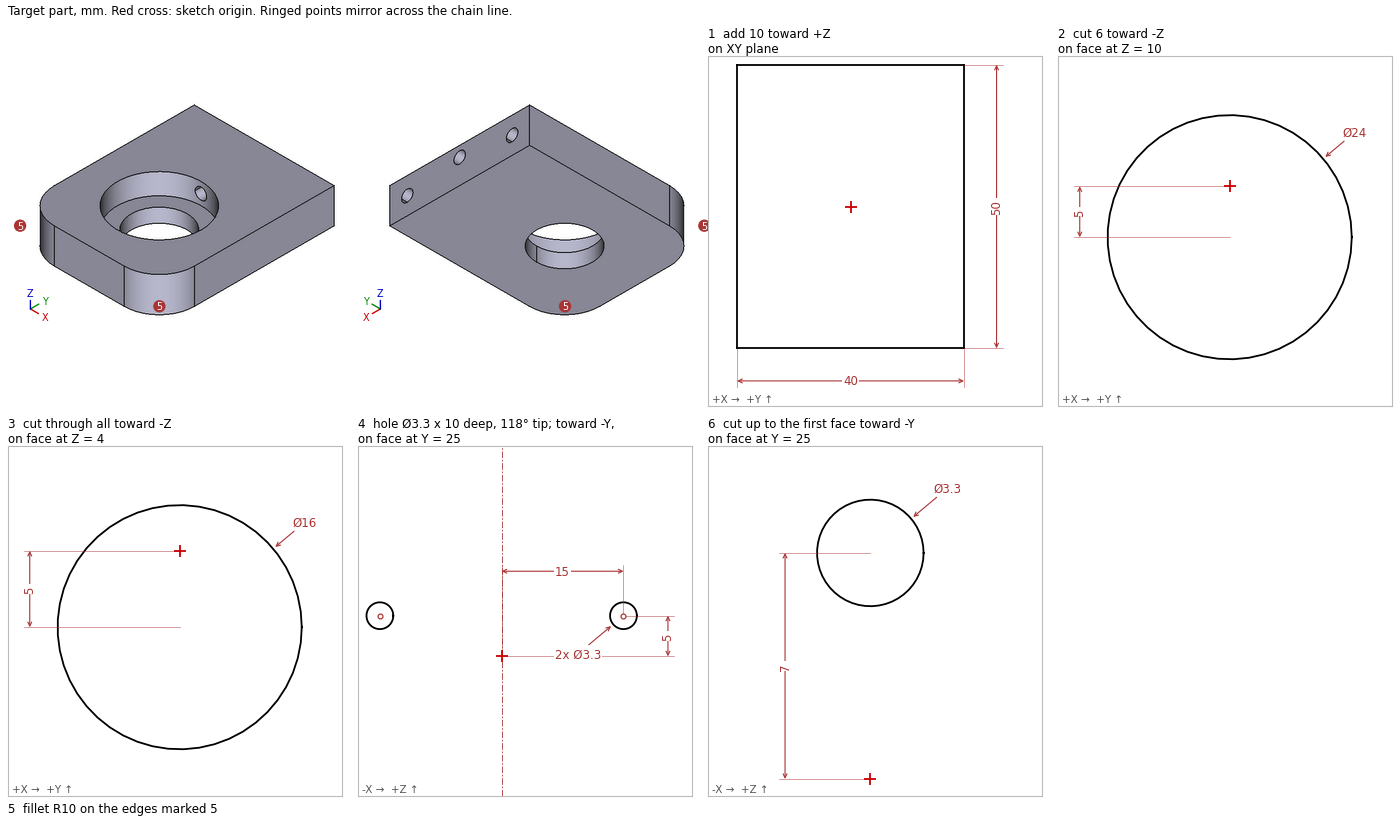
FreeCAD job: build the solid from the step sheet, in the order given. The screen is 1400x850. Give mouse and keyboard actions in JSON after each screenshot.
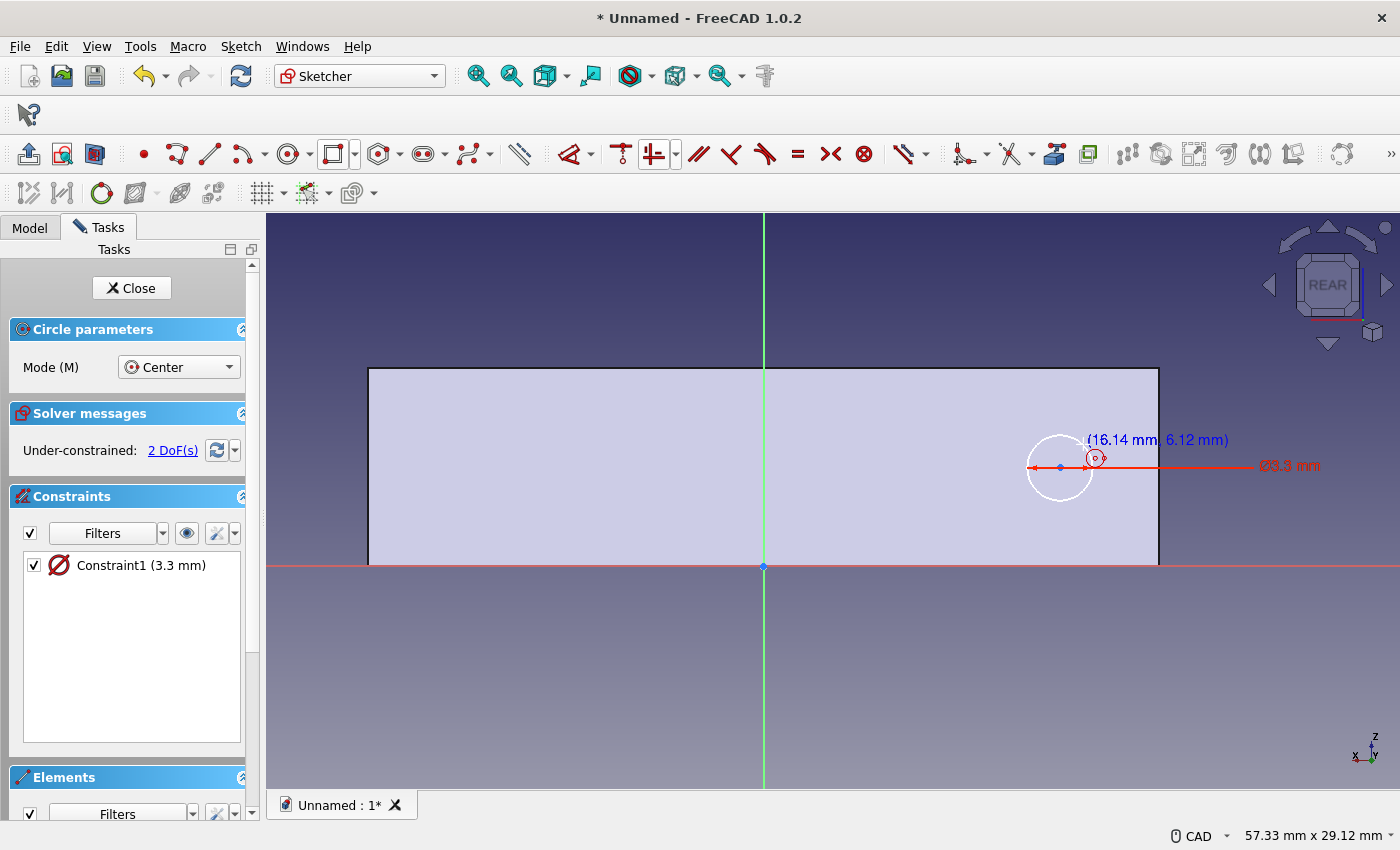
{"action": "left_click", "coordinate": [467, 467]}
{"action": "mouse_move", "coordinate": [490, 444]}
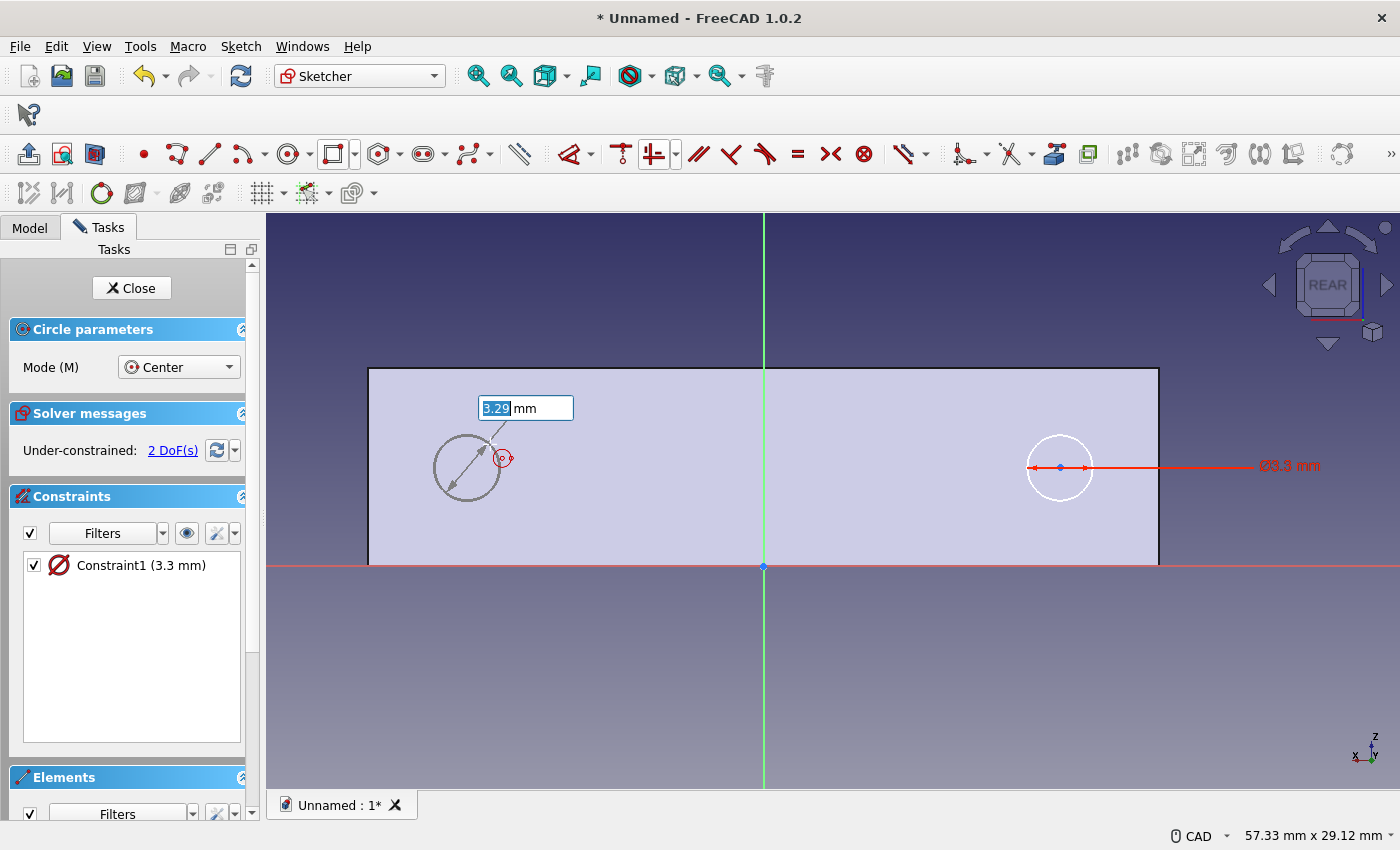
{"action": "type", "text": "3.3"}
{"action": "key", "text": "Return"}
{"action": "key", "text": "Escape"}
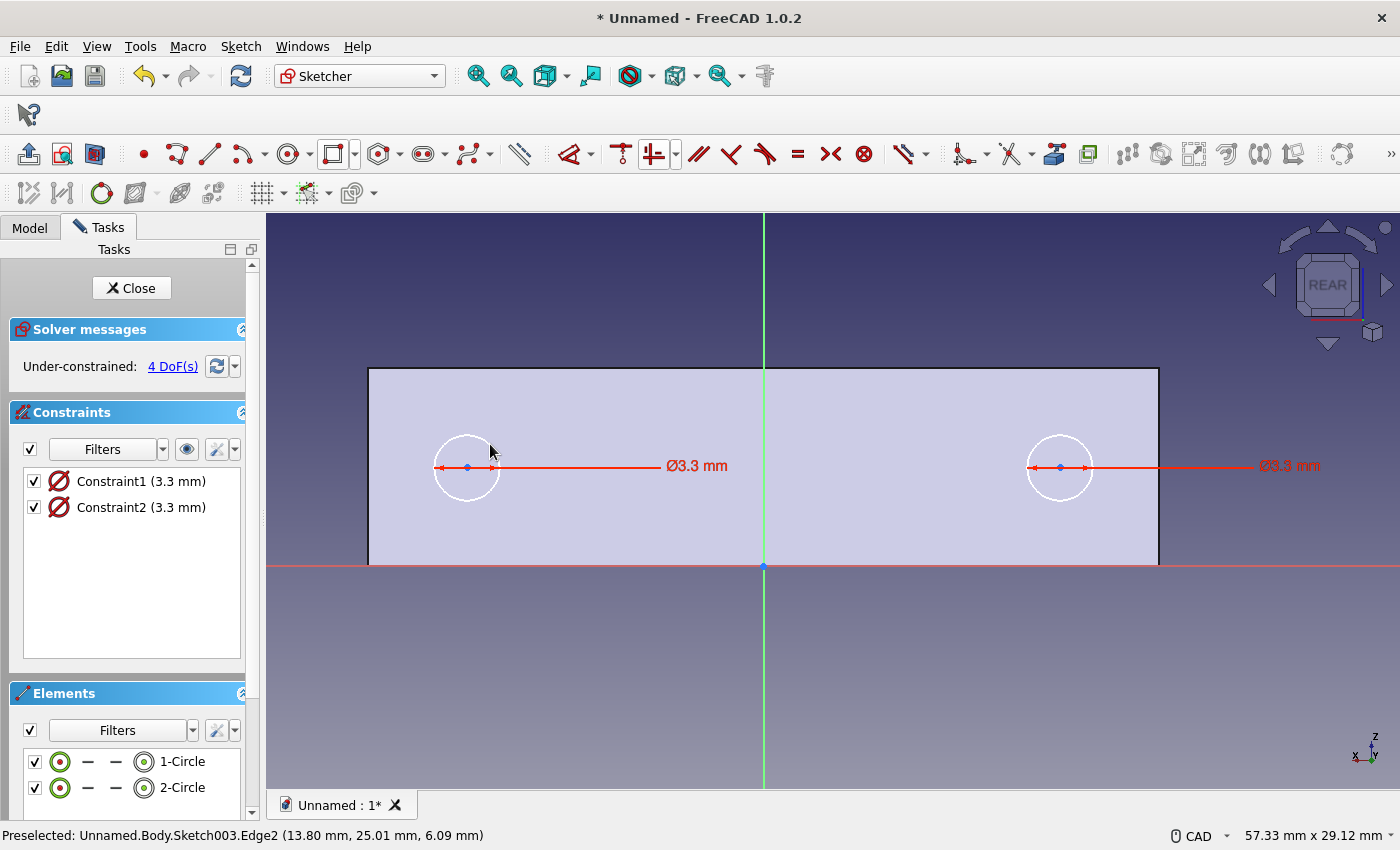
{"action": "left_click", "coordinate": [1060, 468]}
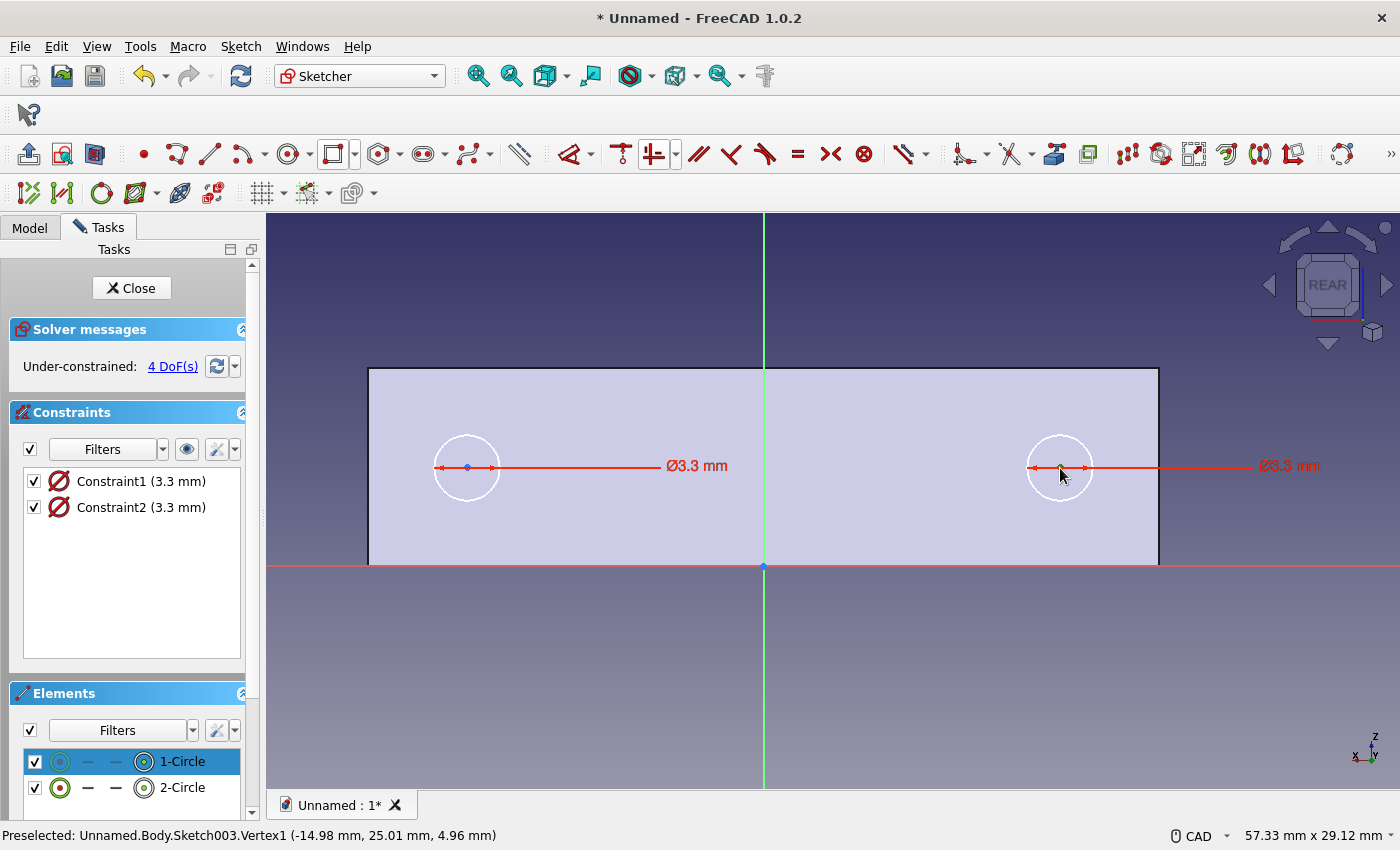
{"action": "left_click", "coordinate": [467, 468]}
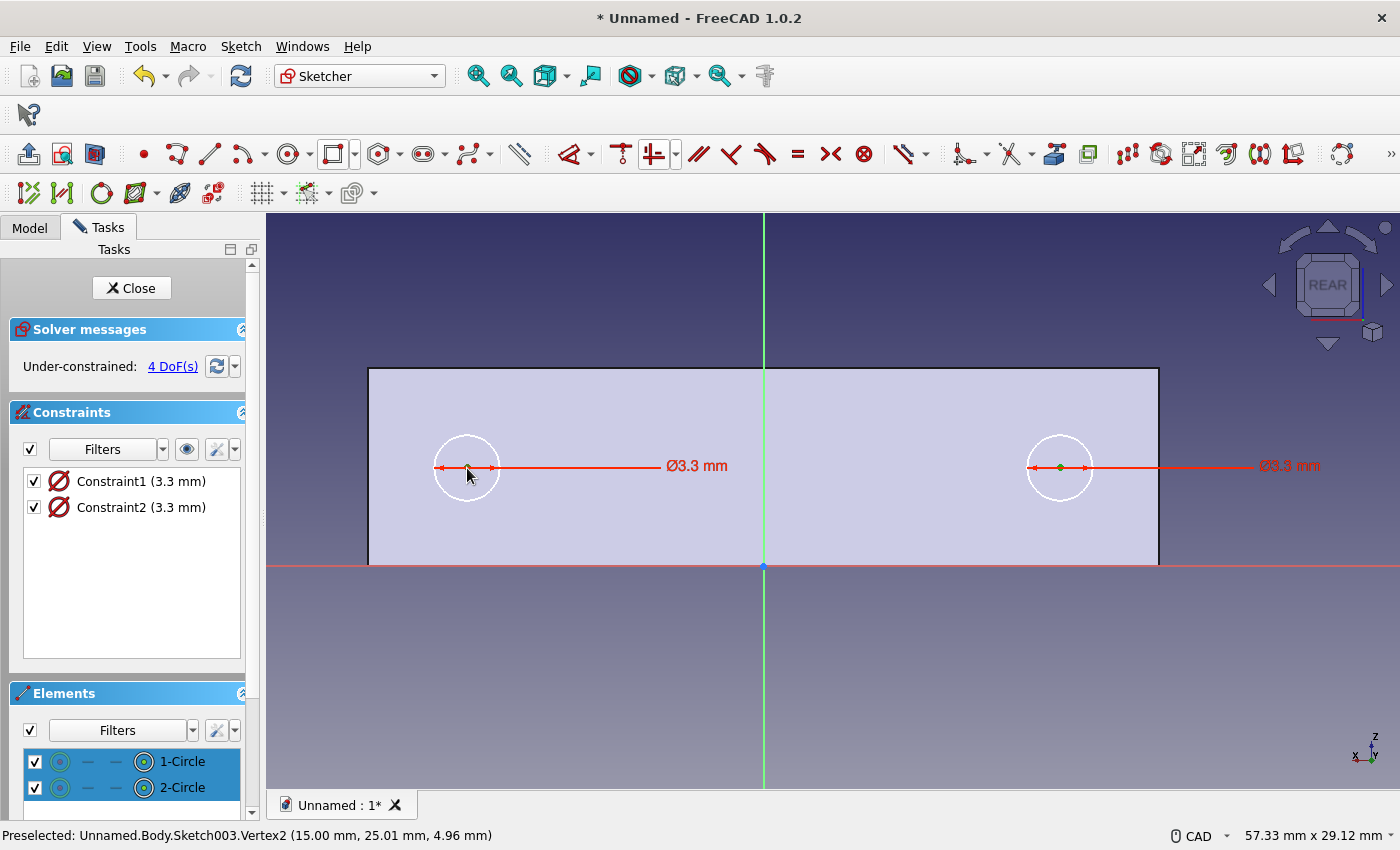
{"action": "left_click", "coordinate": [764, 724]}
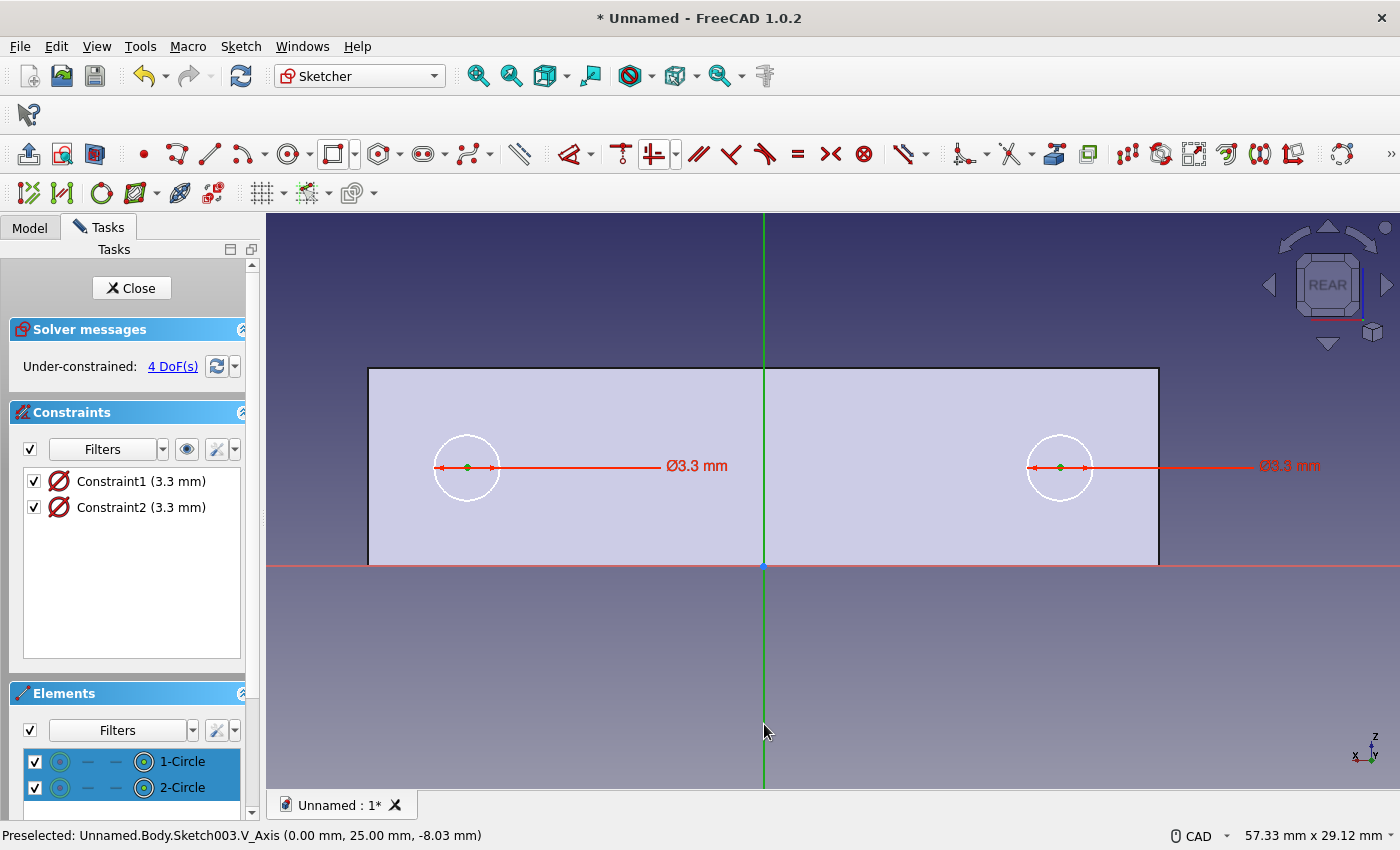
{"action": "left_click", "coordinate": [831, 154]}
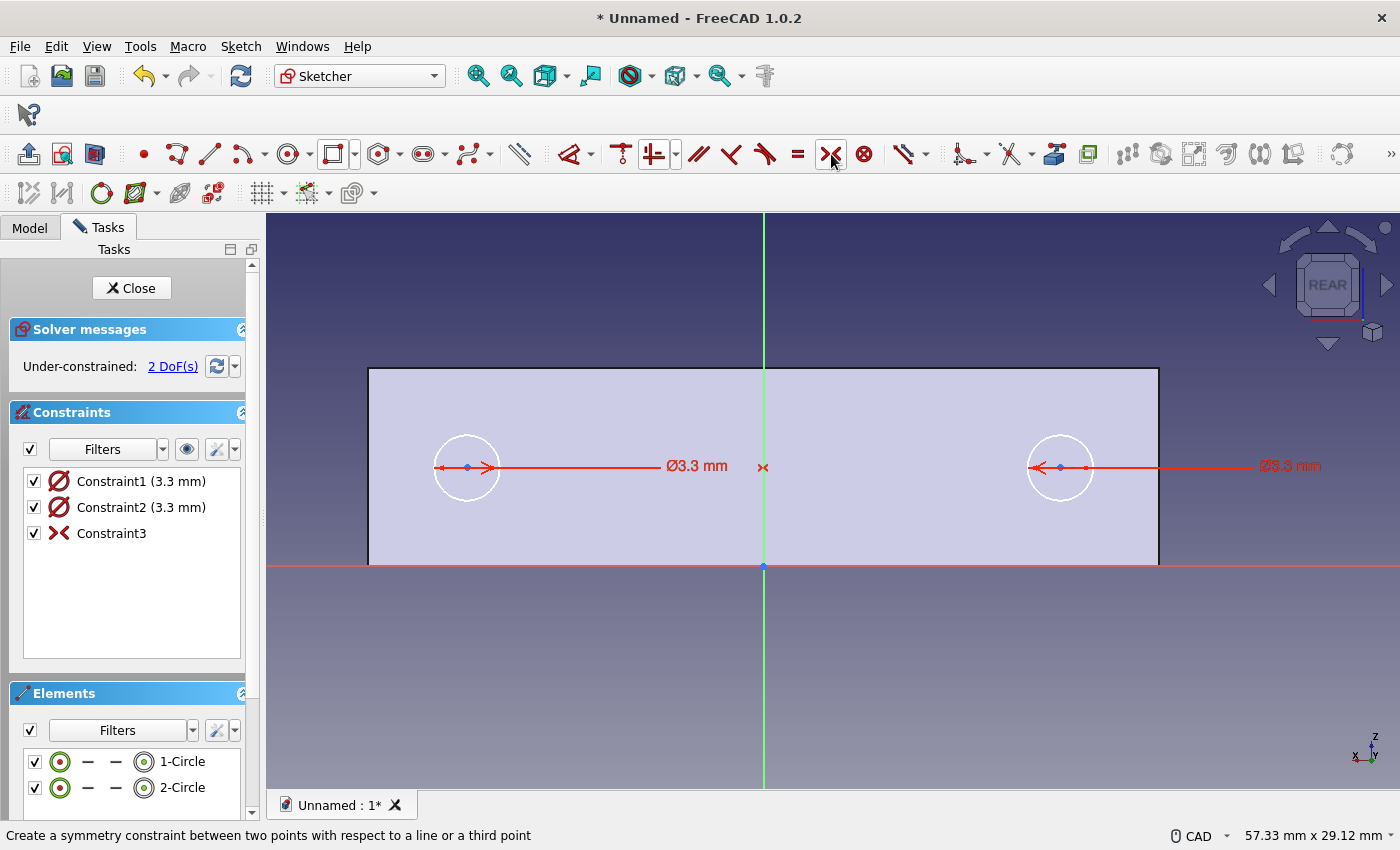
{"action": "left_click", "coordinate": [568, 154]}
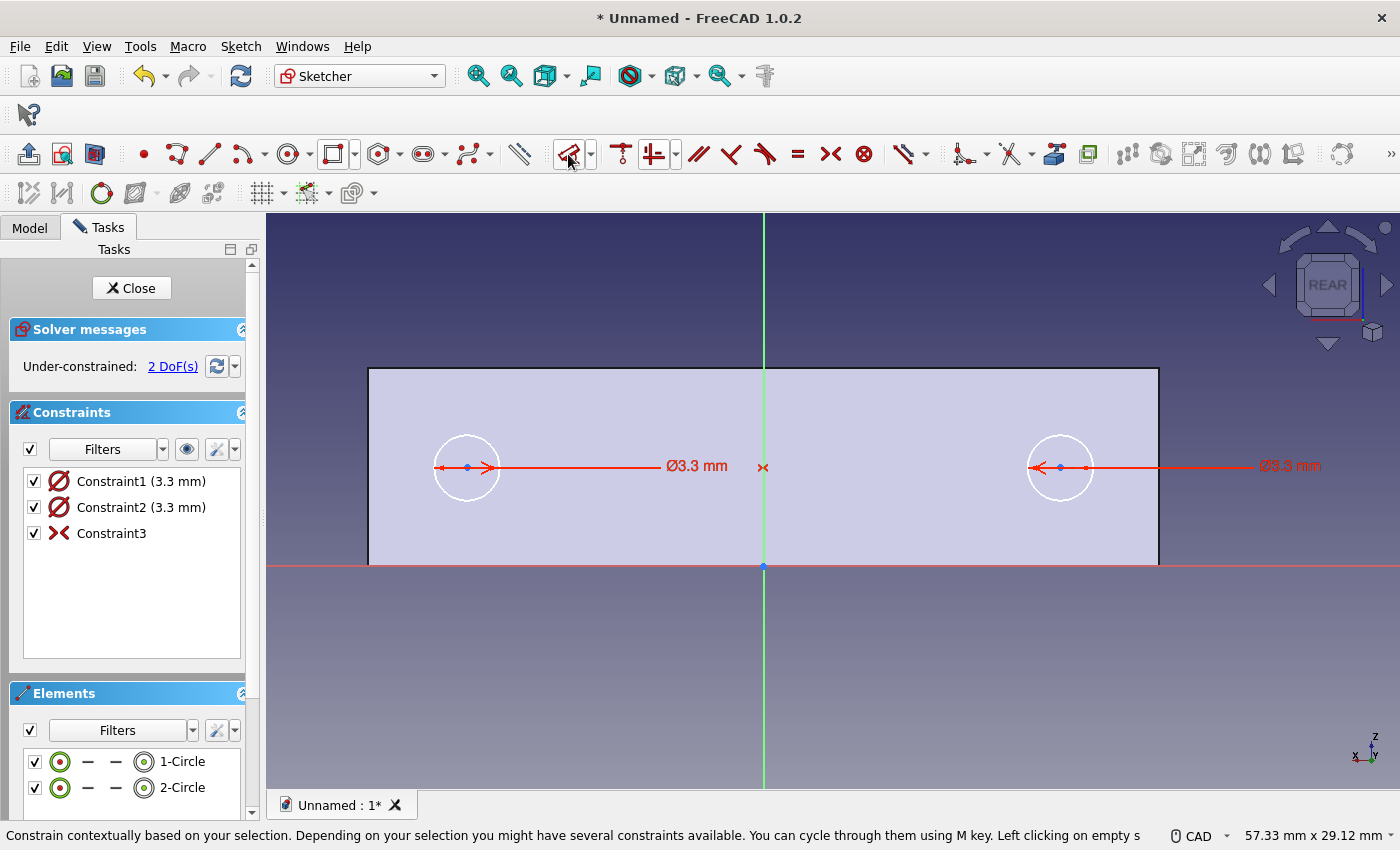
{"action": "left_click", "coordinate": [1060, 468]}
{"action": "left_click", "coordinate": [1094, 517]}